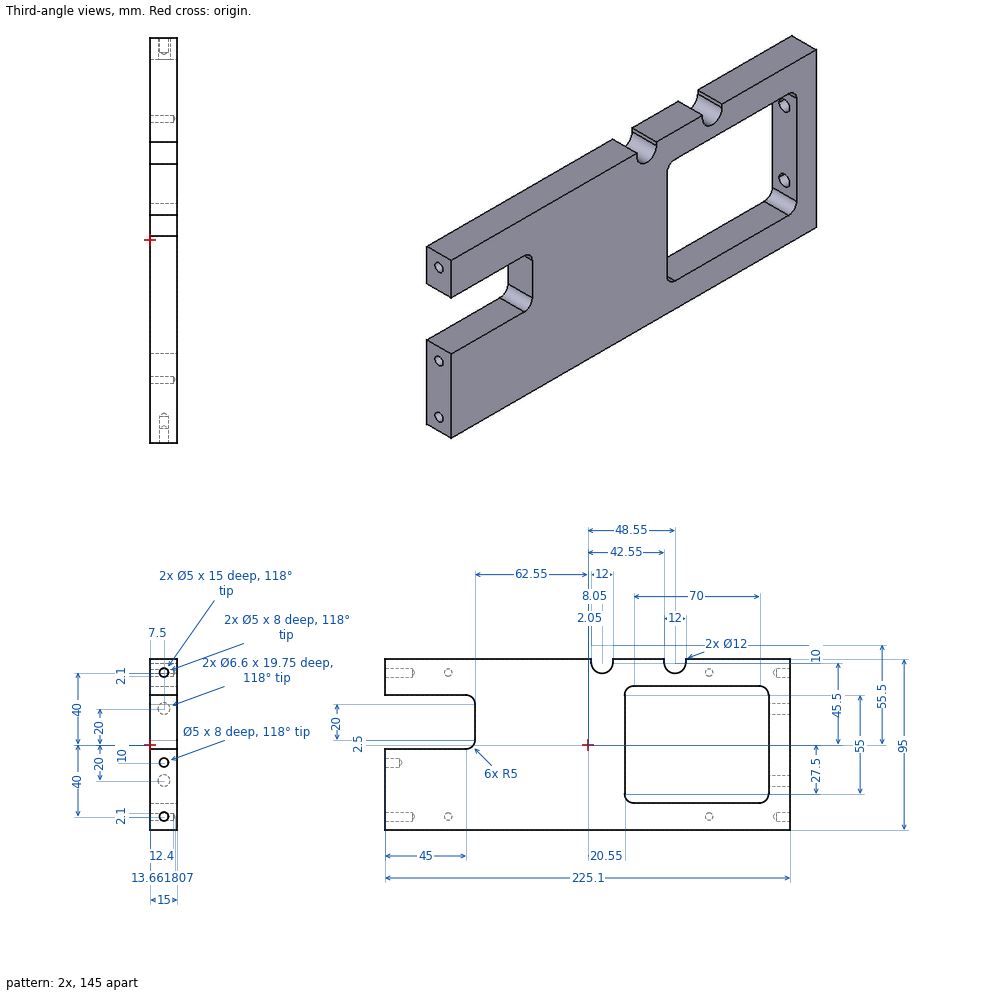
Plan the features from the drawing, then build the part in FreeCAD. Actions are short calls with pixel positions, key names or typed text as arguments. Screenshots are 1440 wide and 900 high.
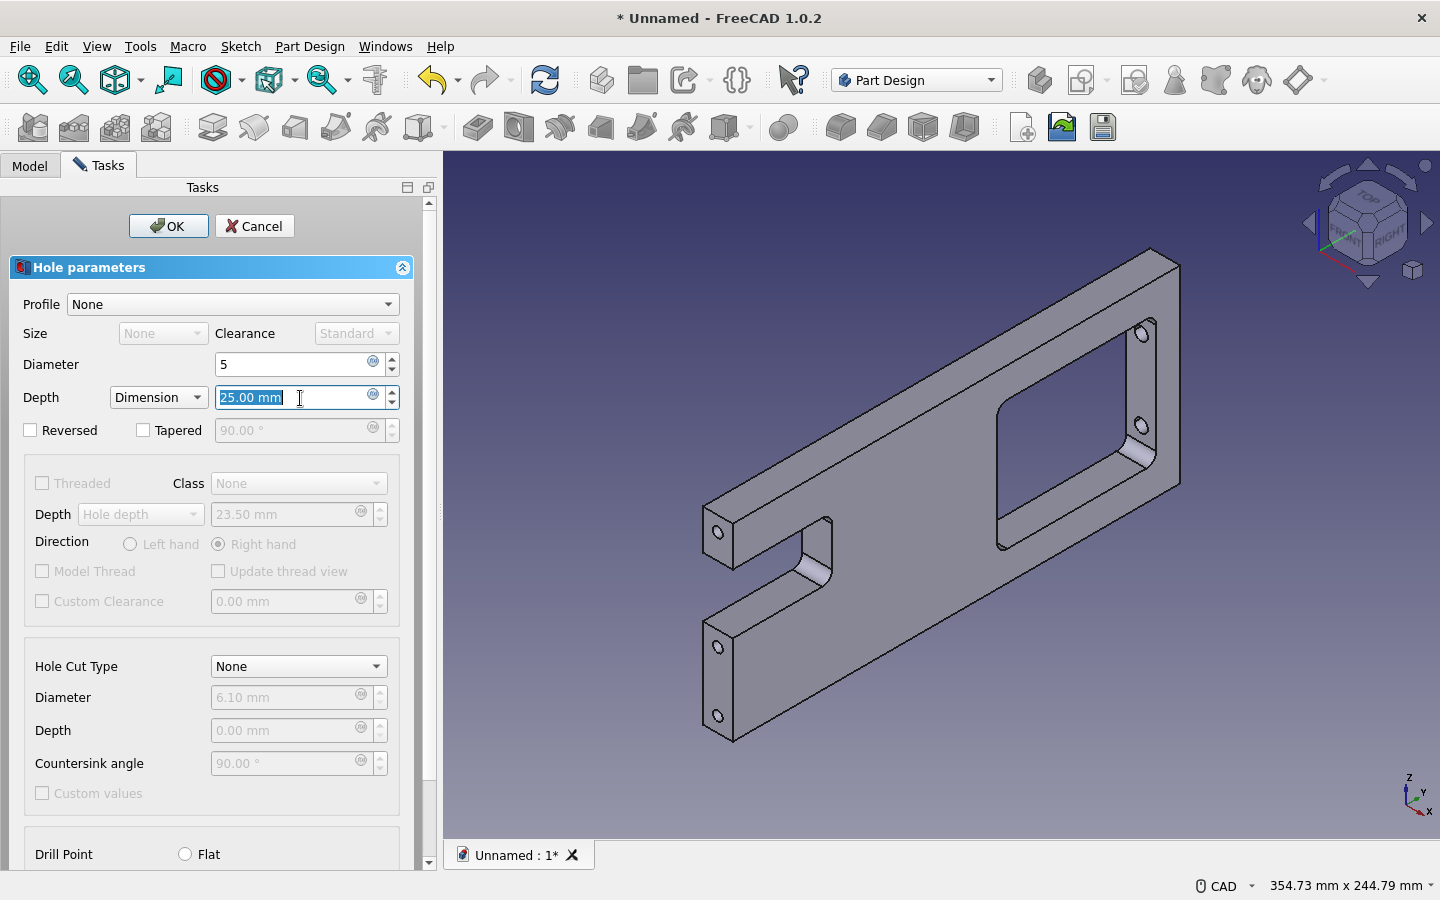
text(8)
key(Tab)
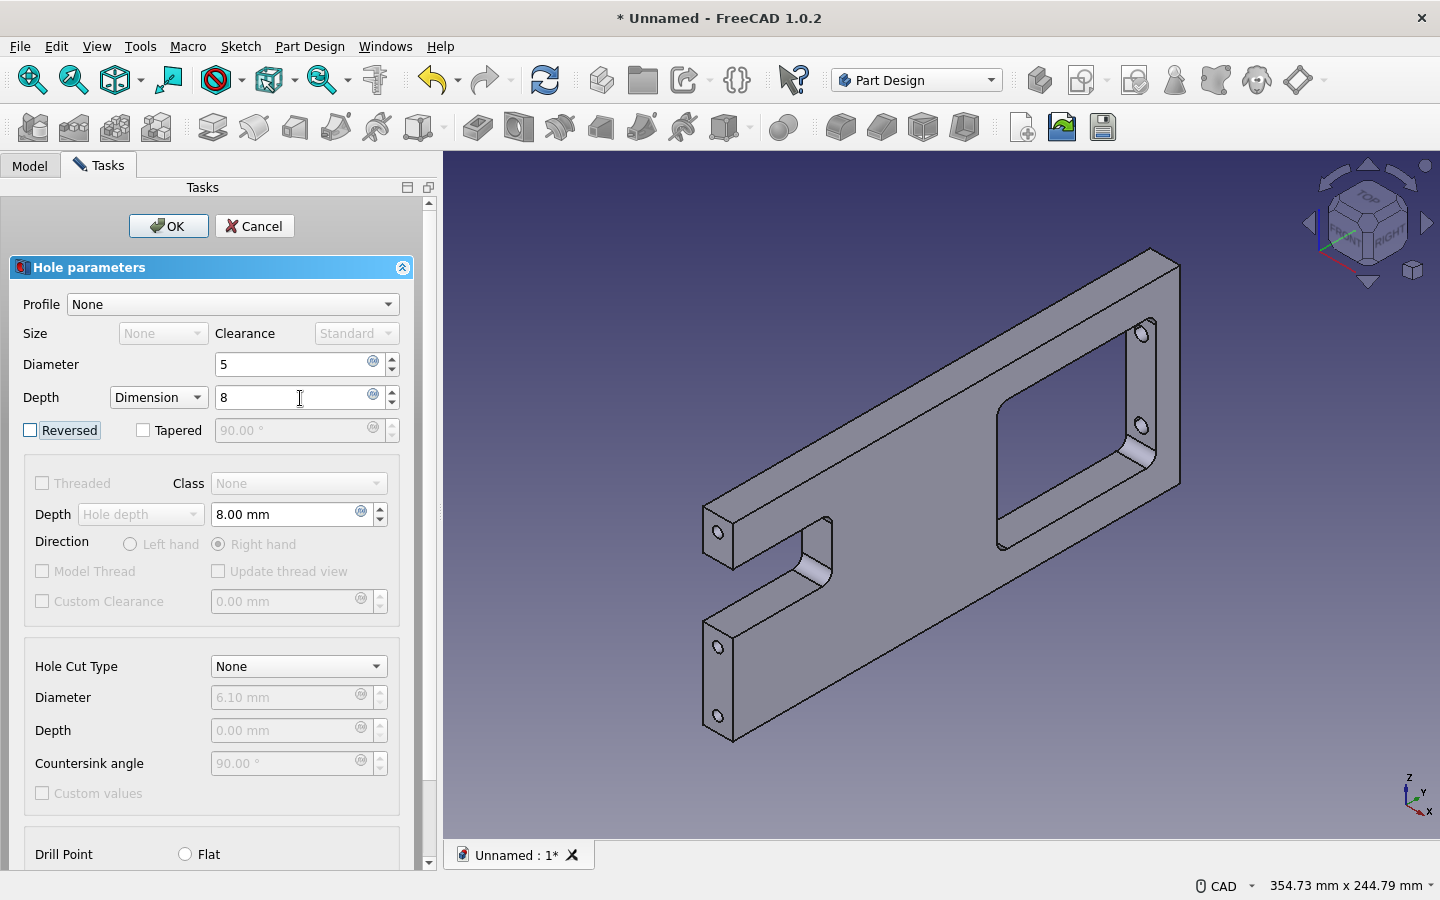
click(169, 226)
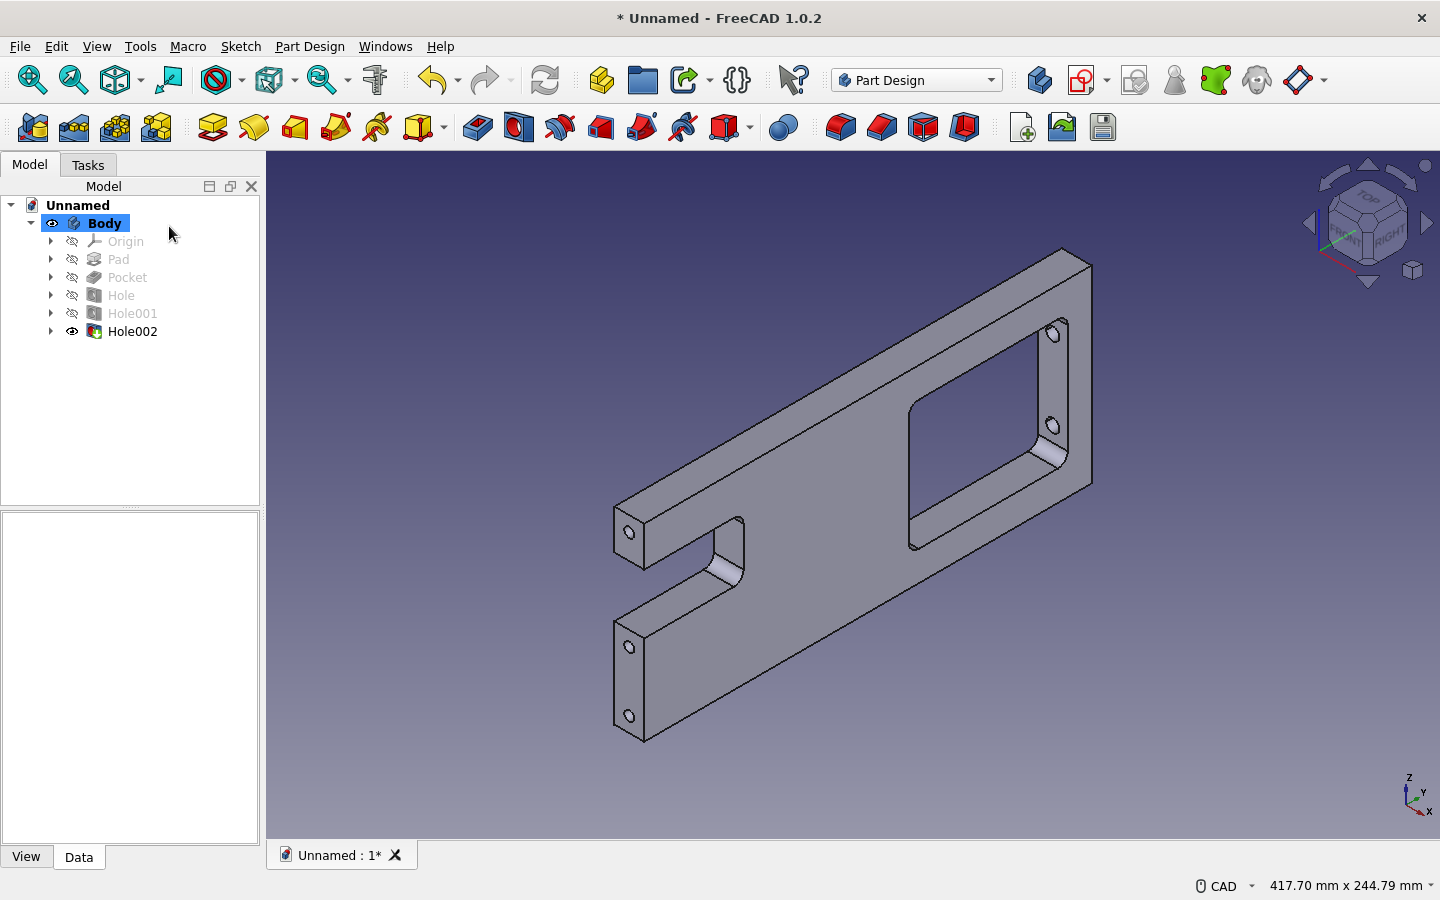
key(4)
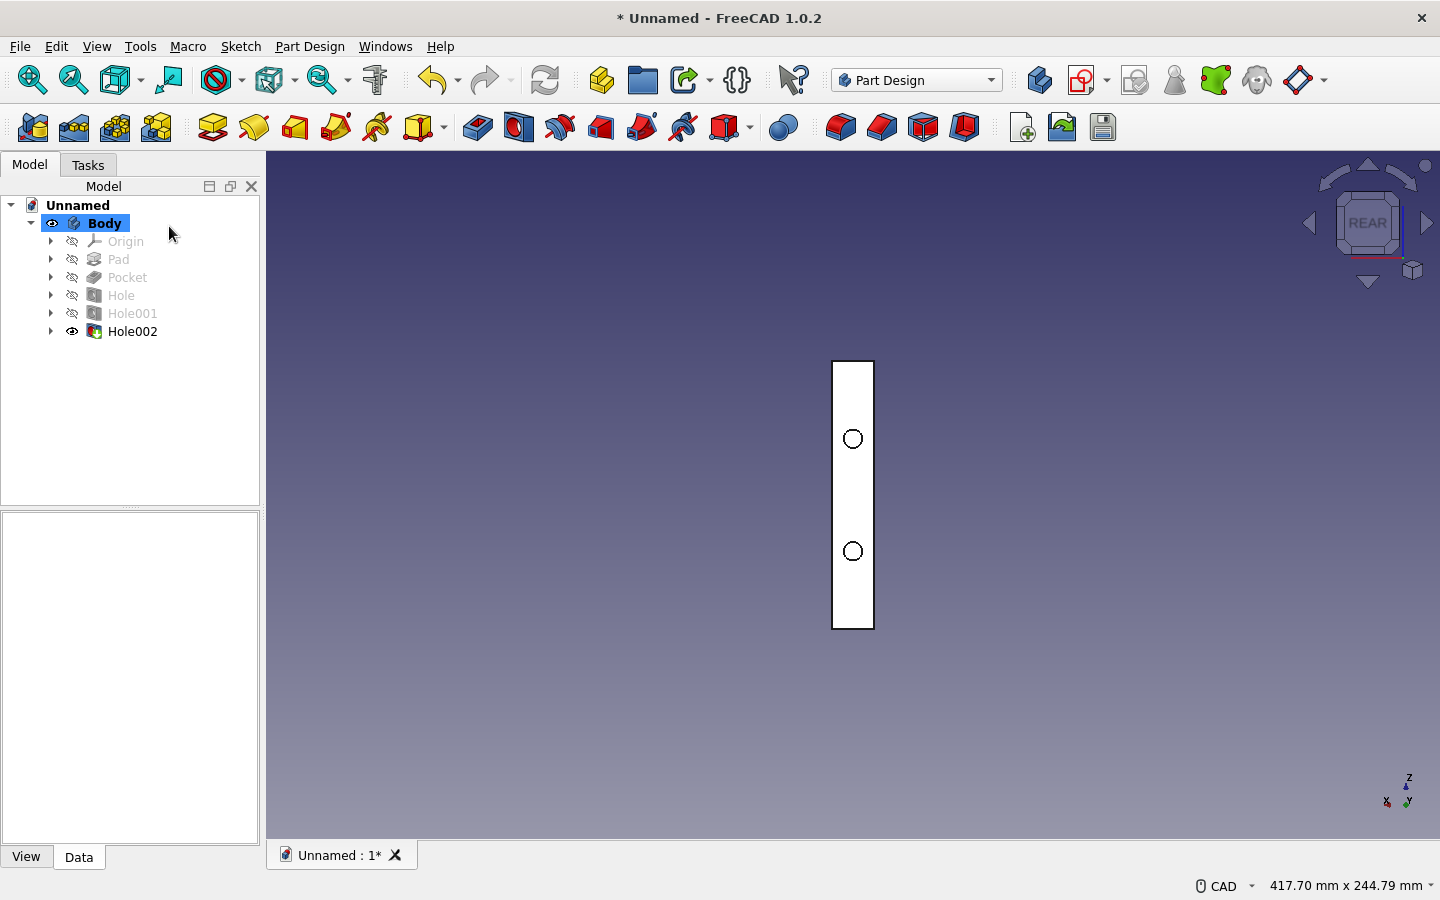
click(33, 80)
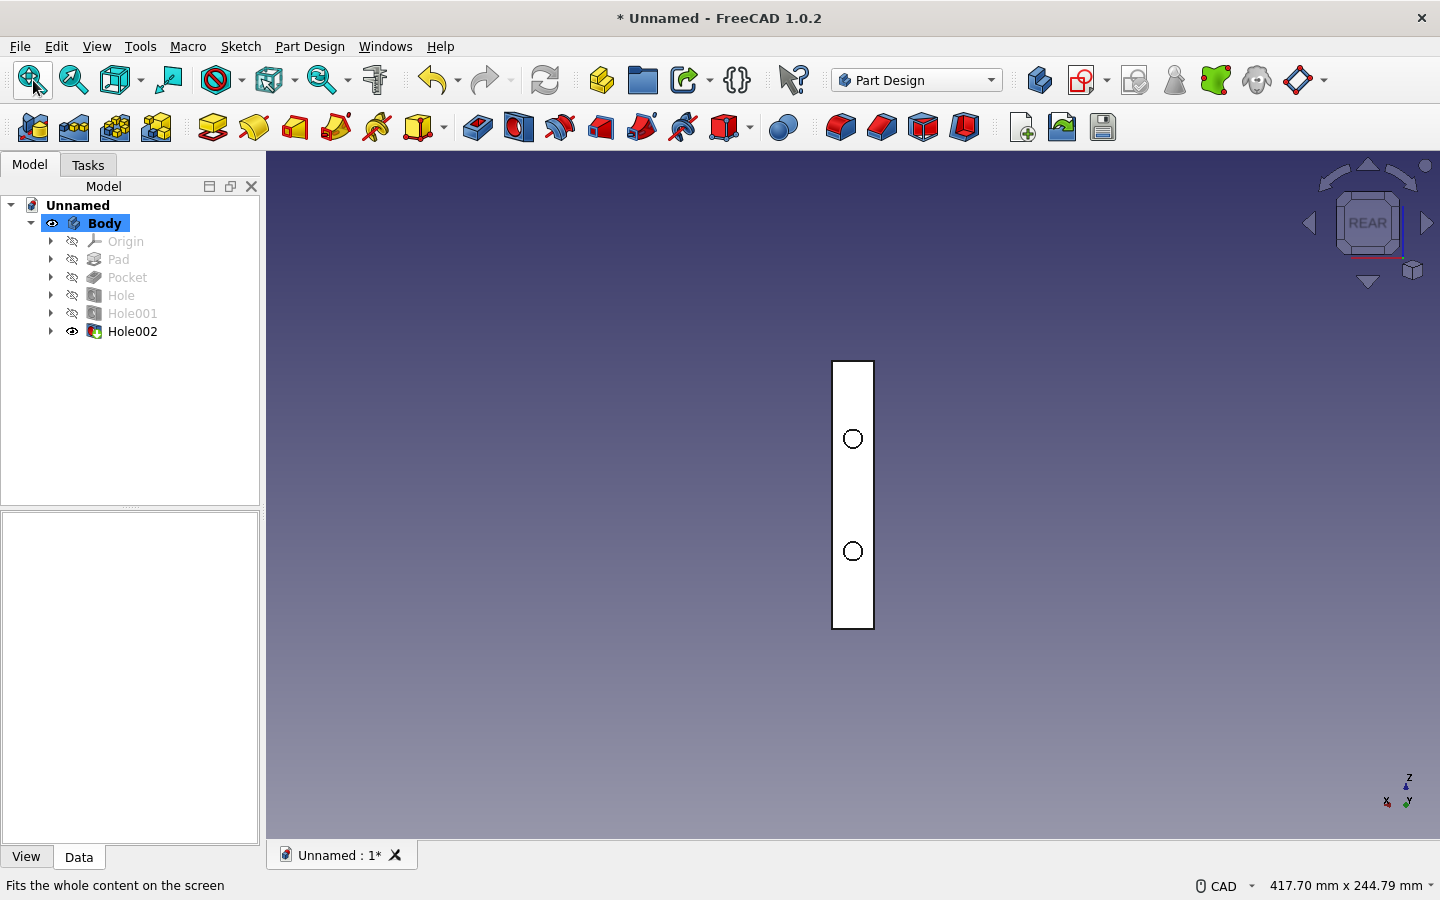
click(853, 494)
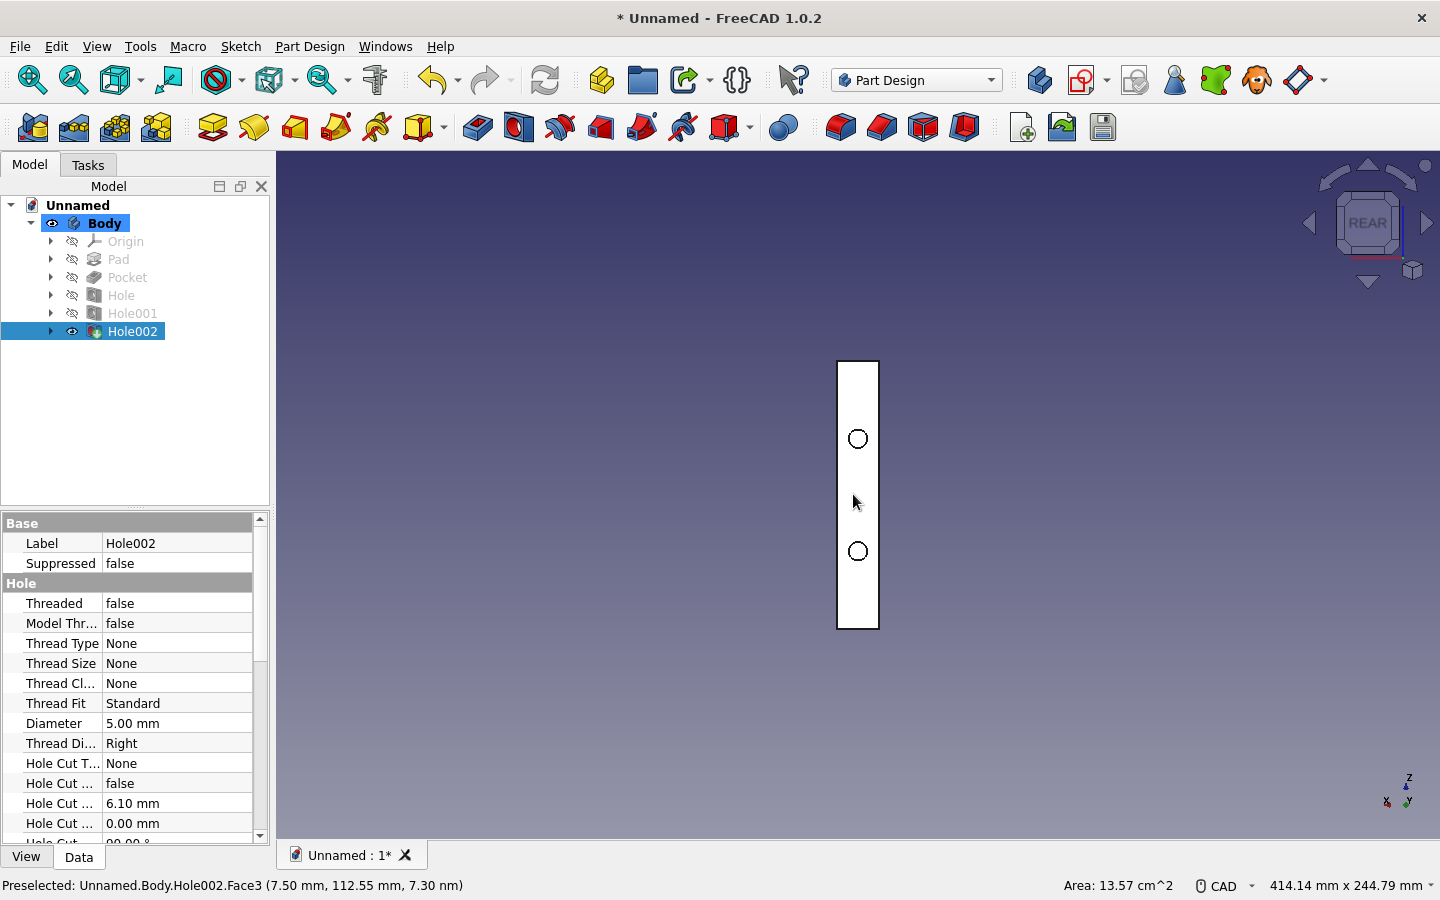
click(1080, 80)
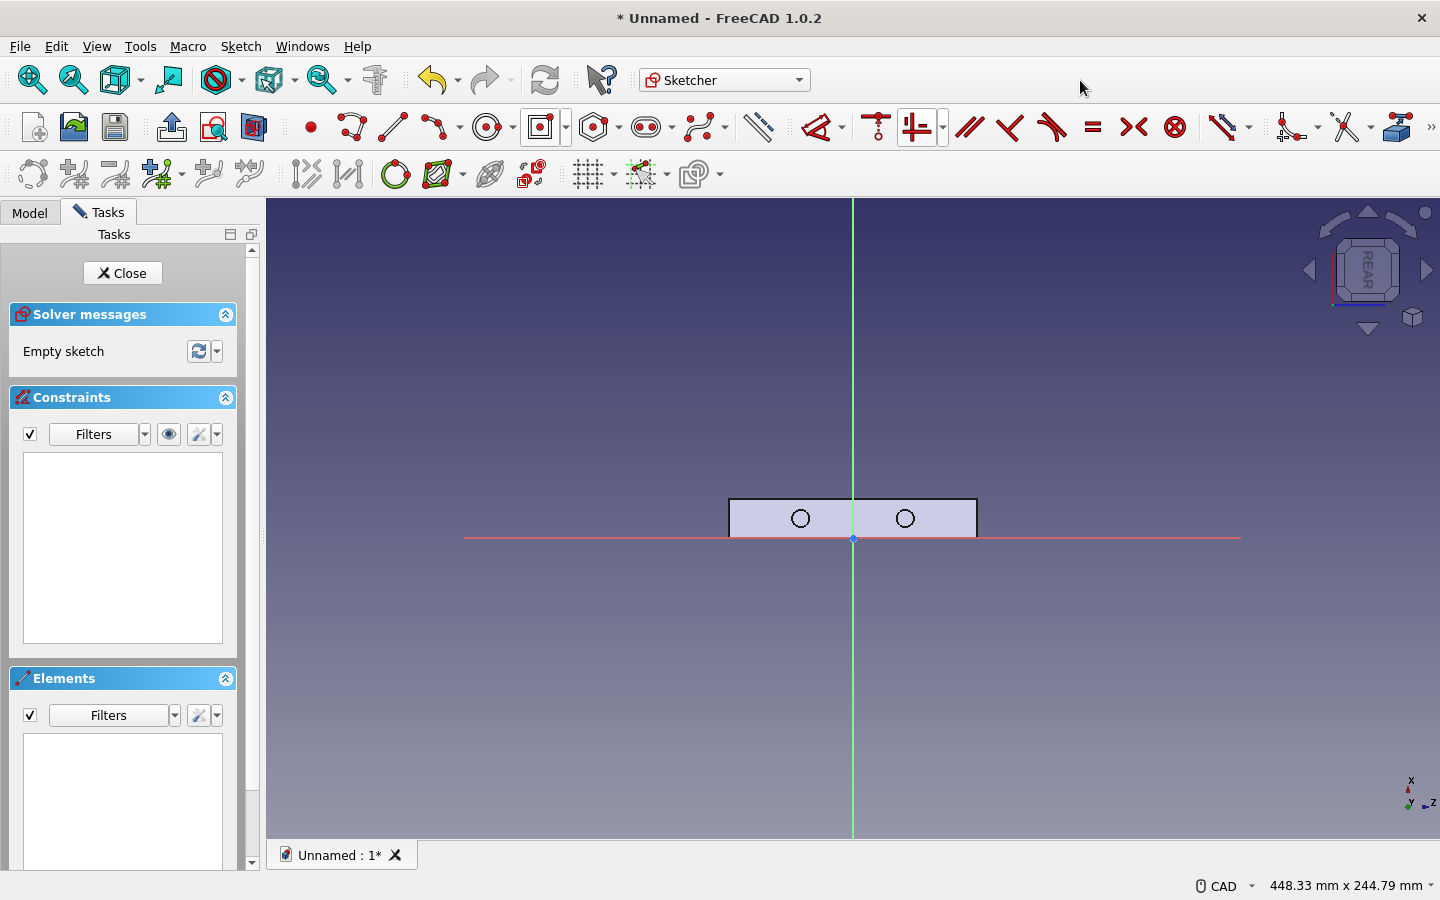
scroll(883, 528, up, 6)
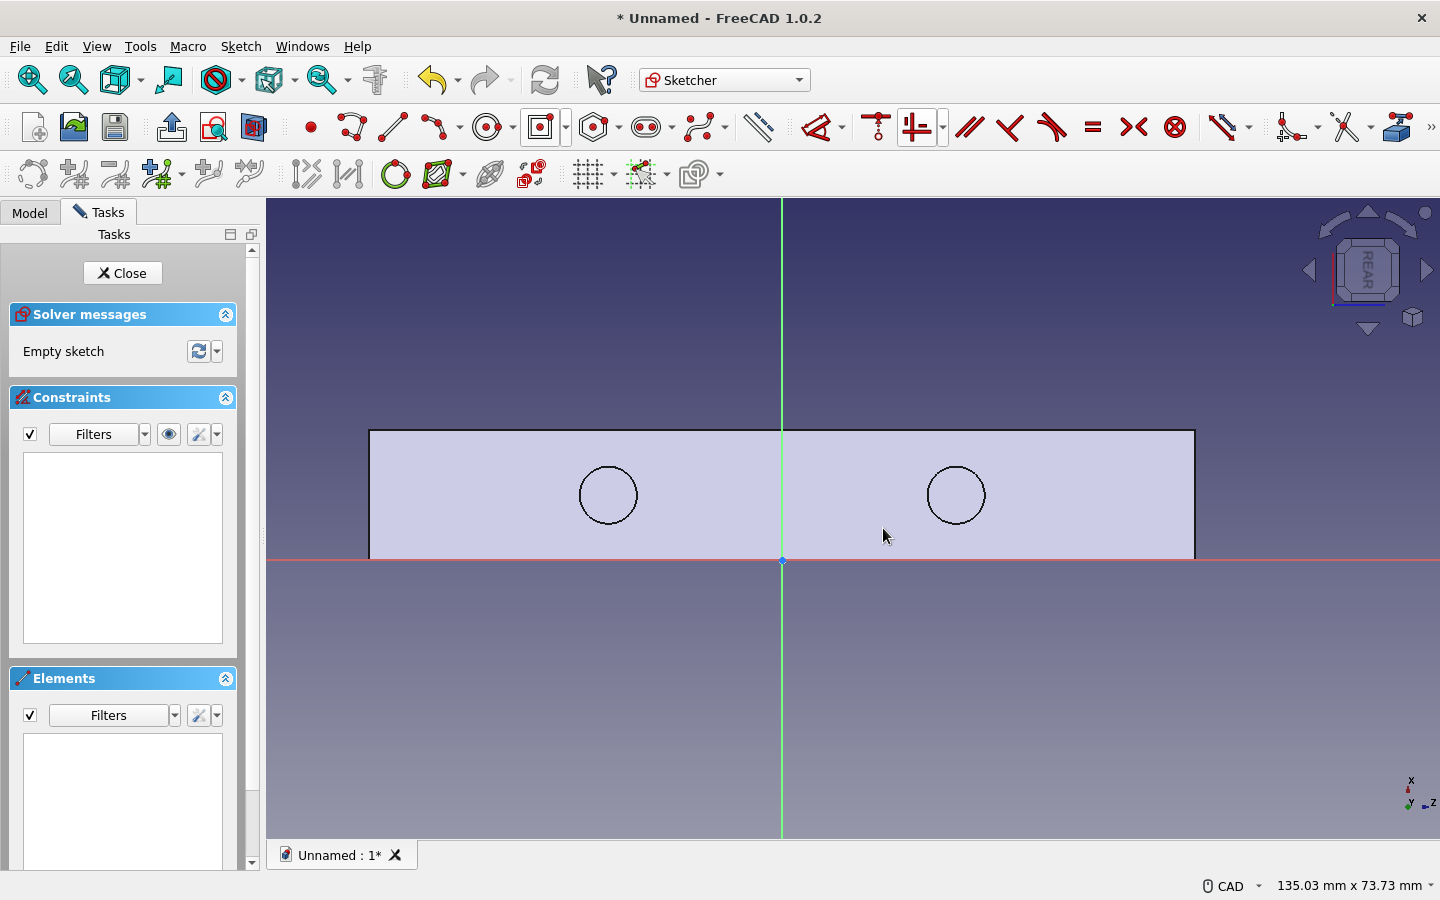
click(486, 128)